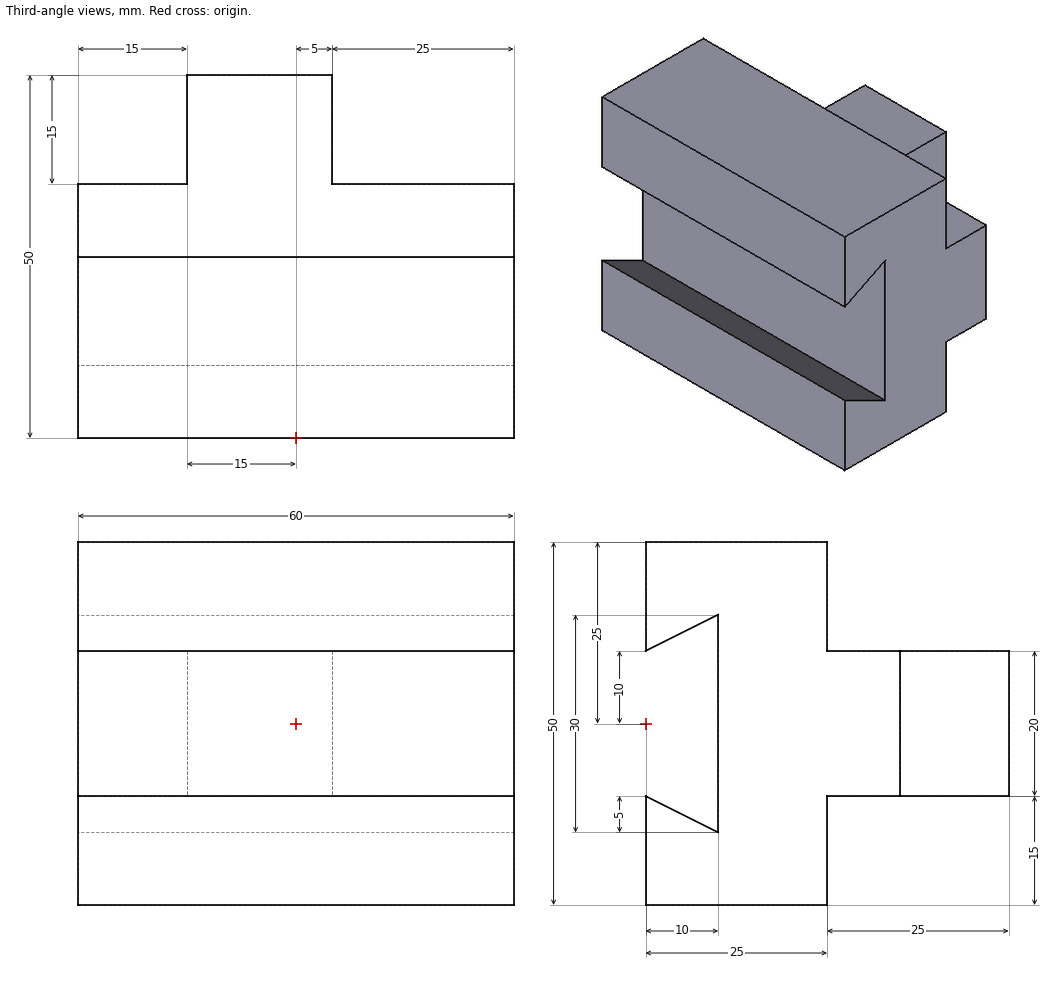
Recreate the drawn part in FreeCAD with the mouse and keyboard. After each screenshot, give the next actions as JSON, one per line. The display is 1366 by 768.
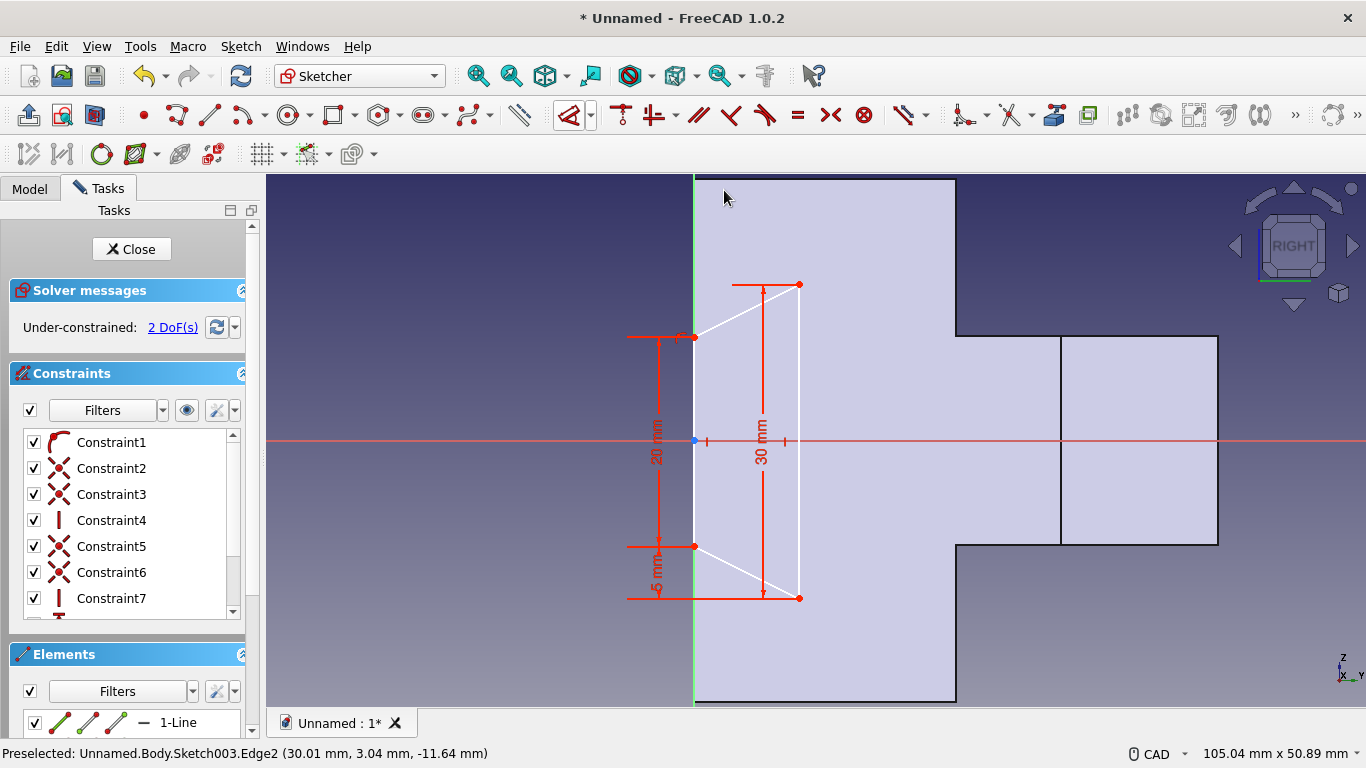
{"action": "left_click", "coordinate": [694, 337]}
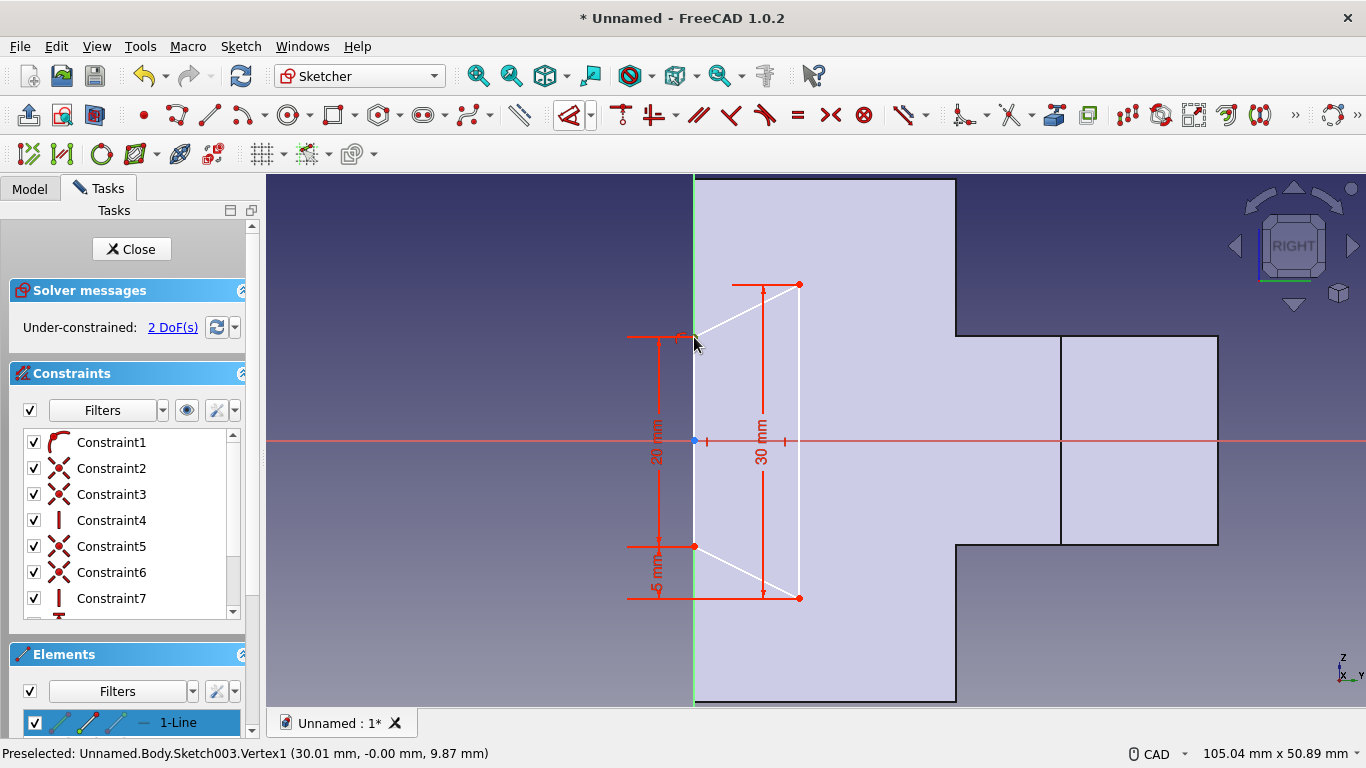
{"action": "key", "text": "i"}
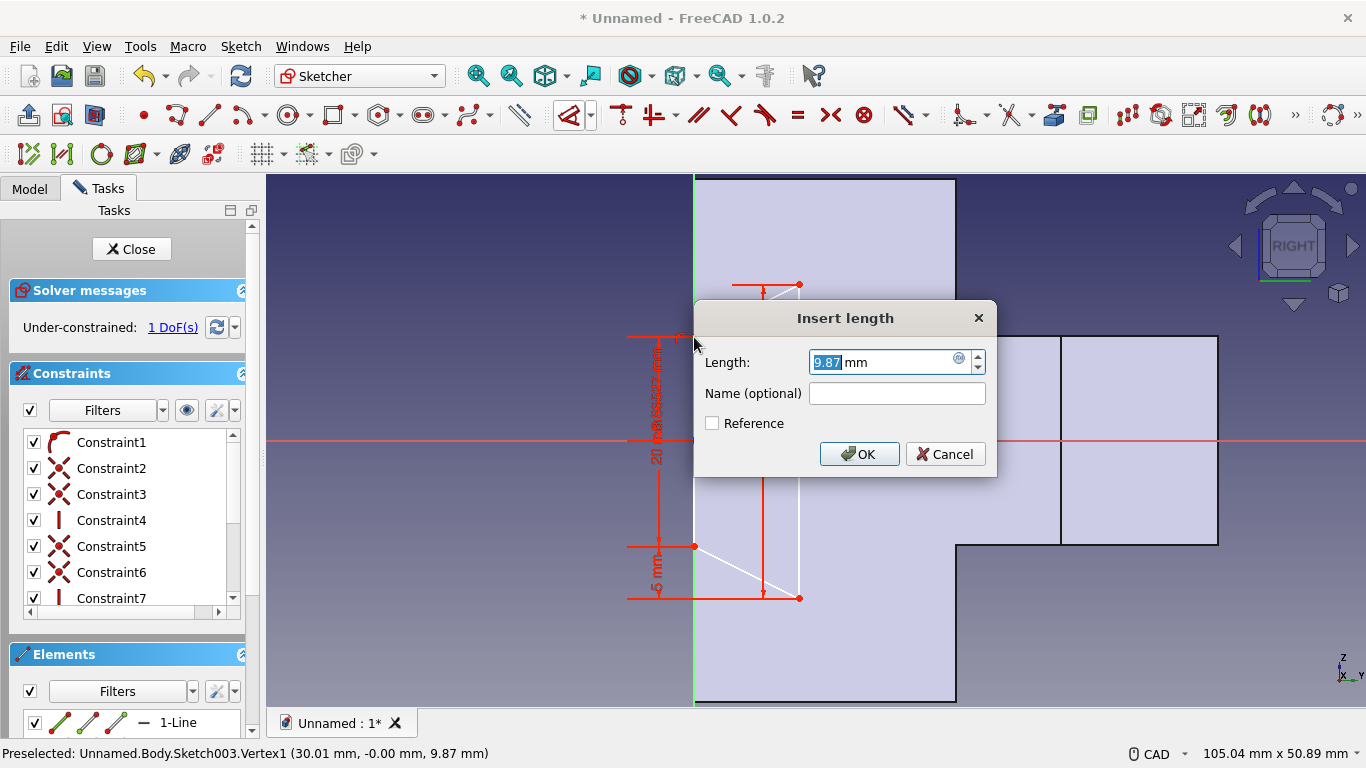
{"action": "type", "text": "10"}
{"action": "key", "text": "Return"}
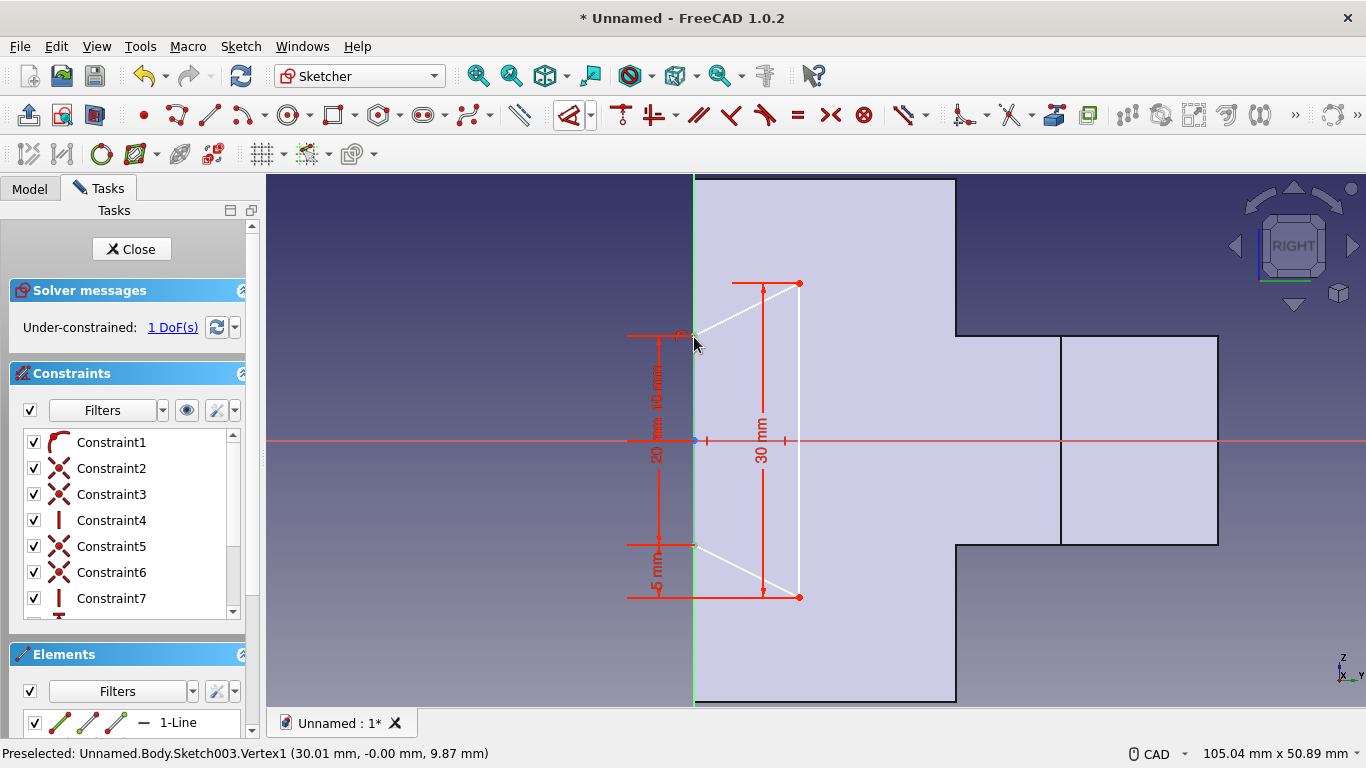
{"action": "left_click", "coordinate": [799, 598]}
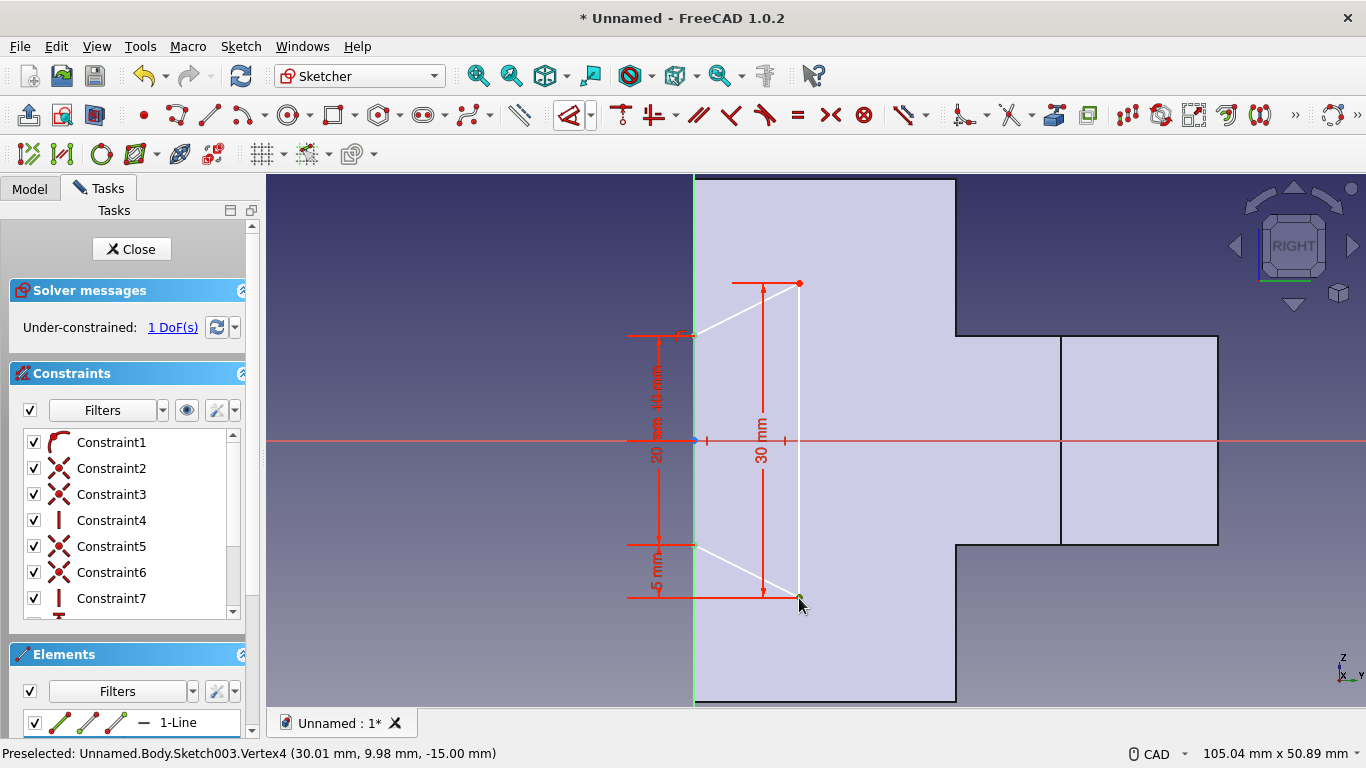
{"action": "key", "text": "l"}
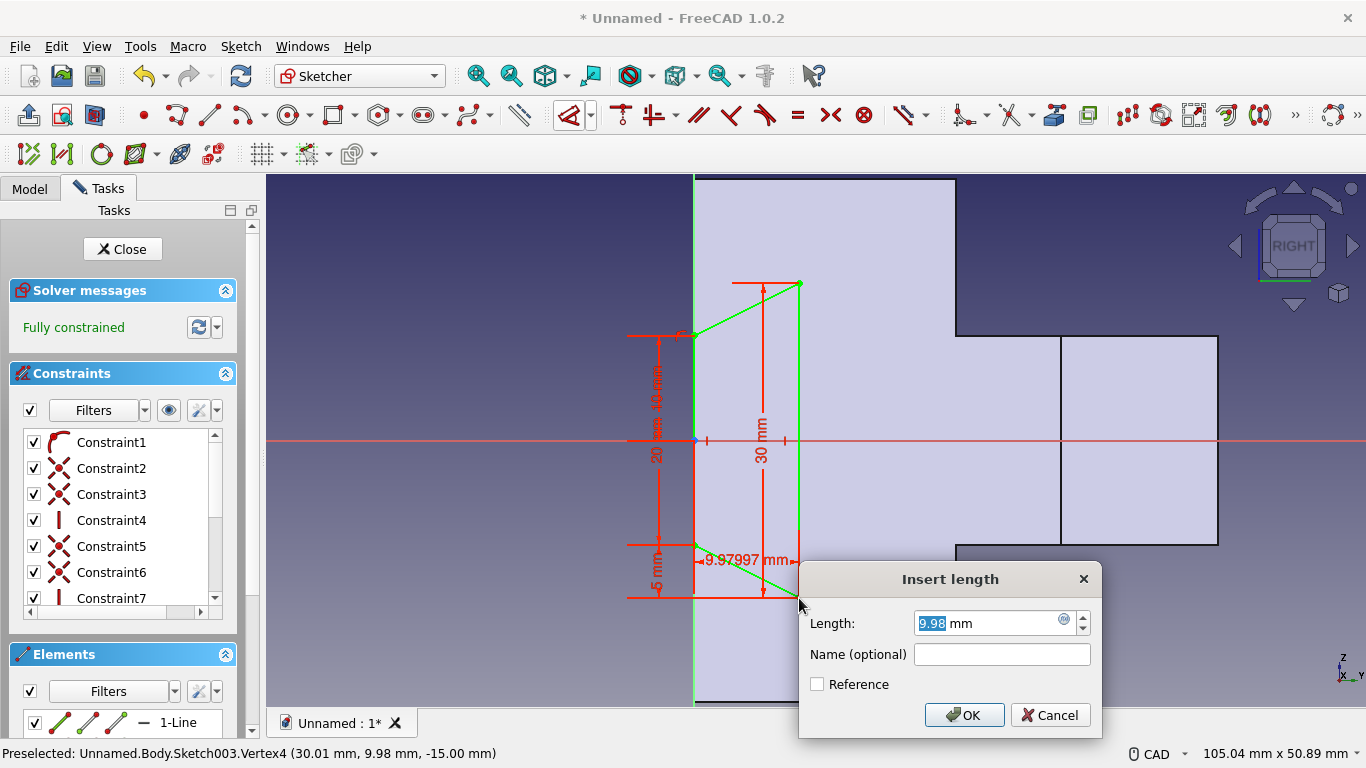
{"action": "type", "text": "10"}
{"action": "key", "text": "Return"}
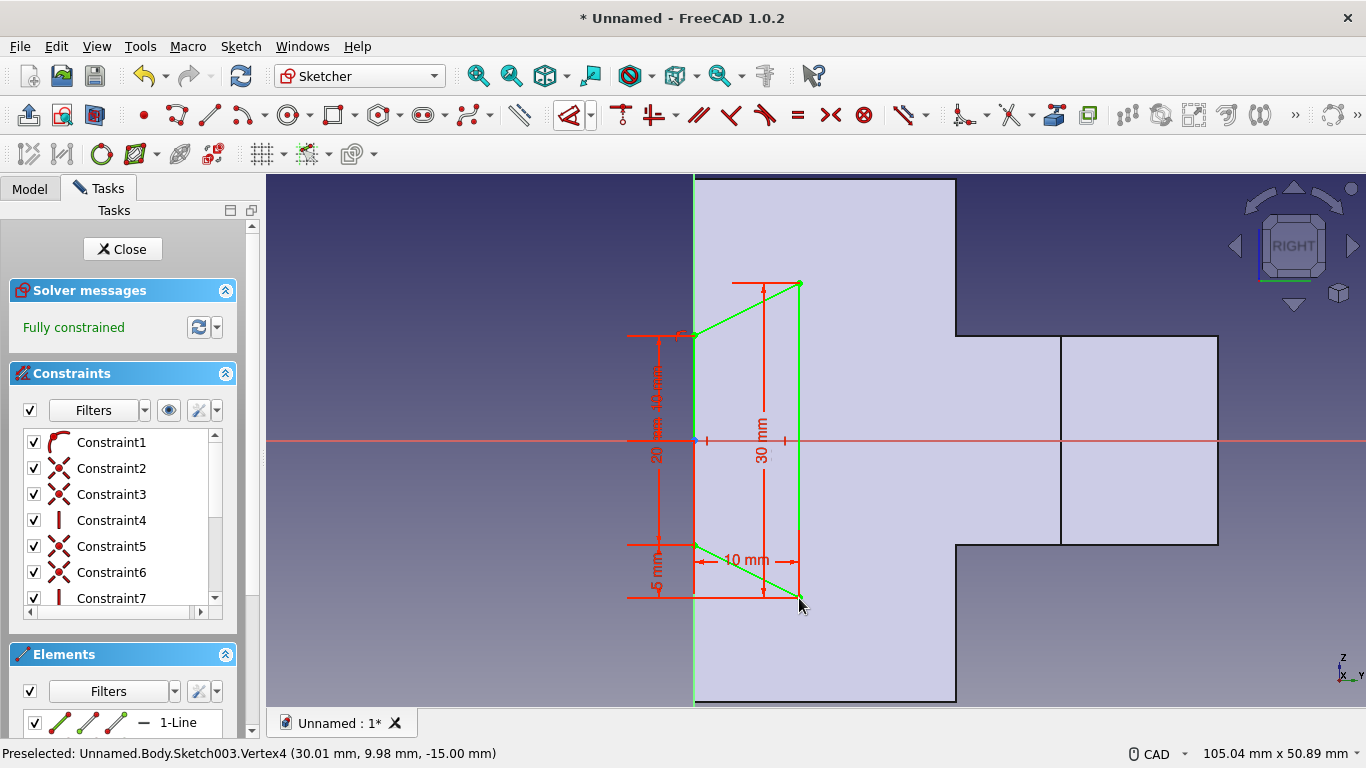
{"action": "left_click", "coordinate": [123, 249]}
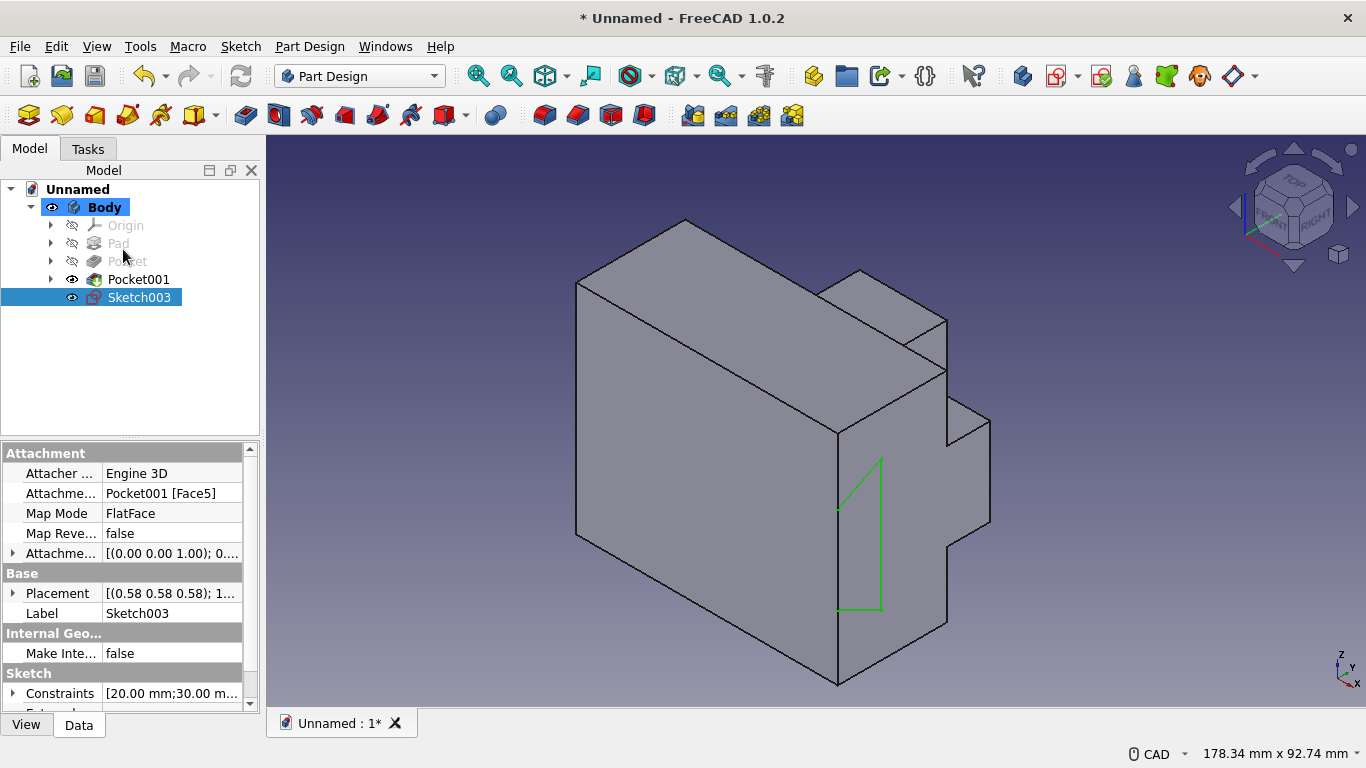
{"action": "left_click", "coordinate": [246, 116]}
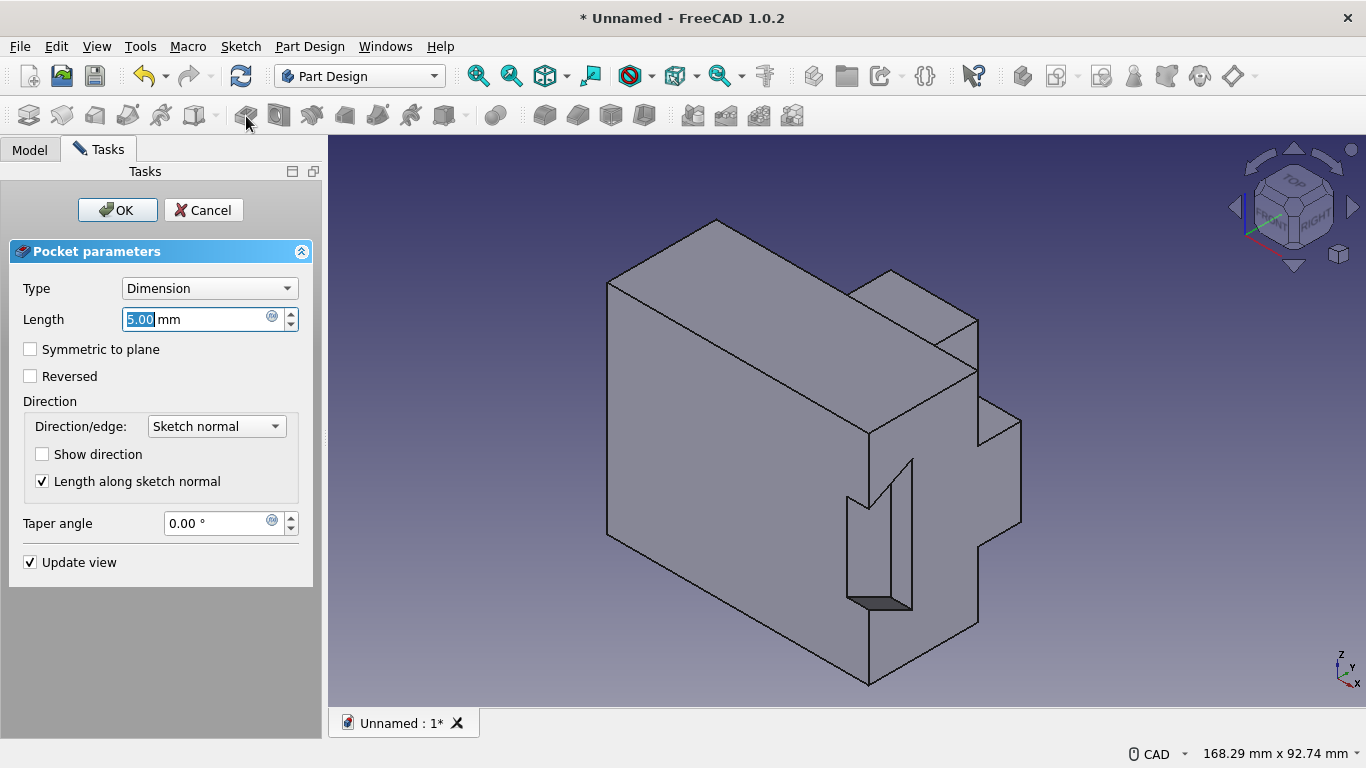
{"action": "left_click", "coordinate": [210, 288]}